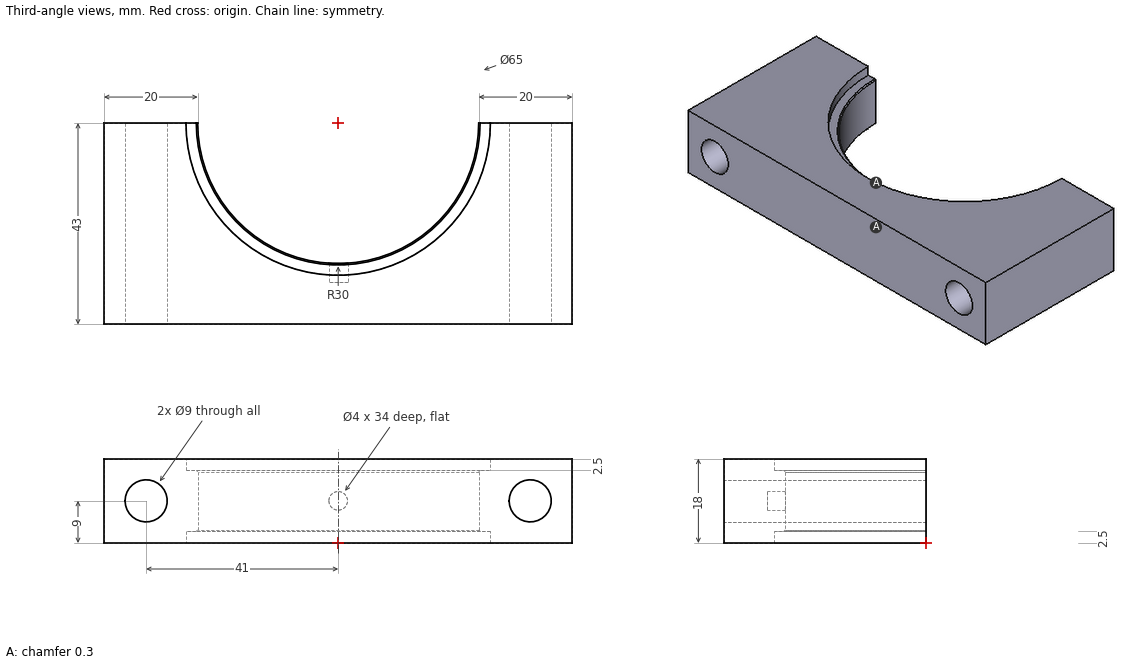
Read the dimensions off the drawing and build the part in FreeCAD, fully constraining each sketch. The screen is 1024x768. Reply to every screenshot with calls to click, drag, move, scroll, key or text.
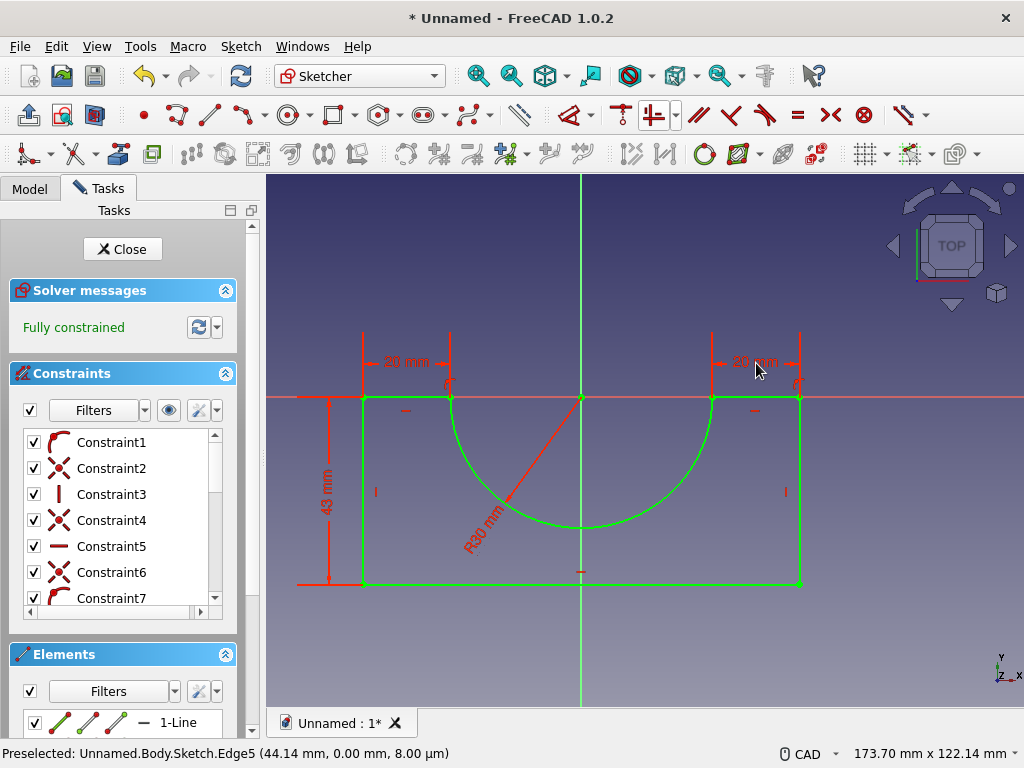
click(123, 249)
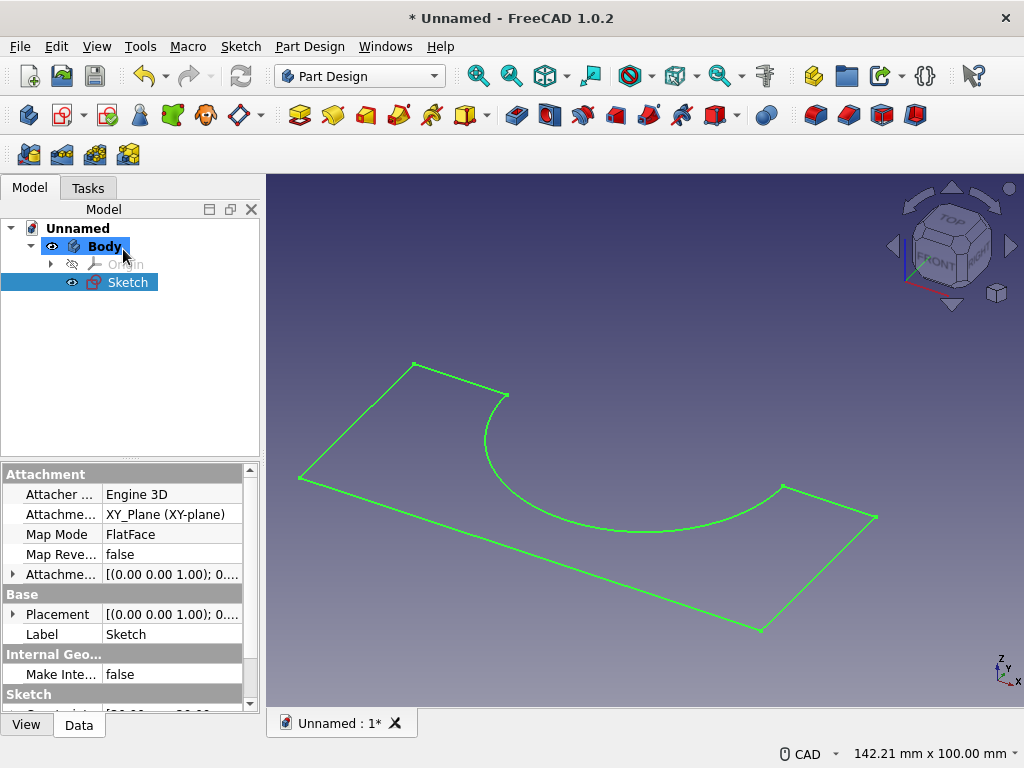
click(300, 116)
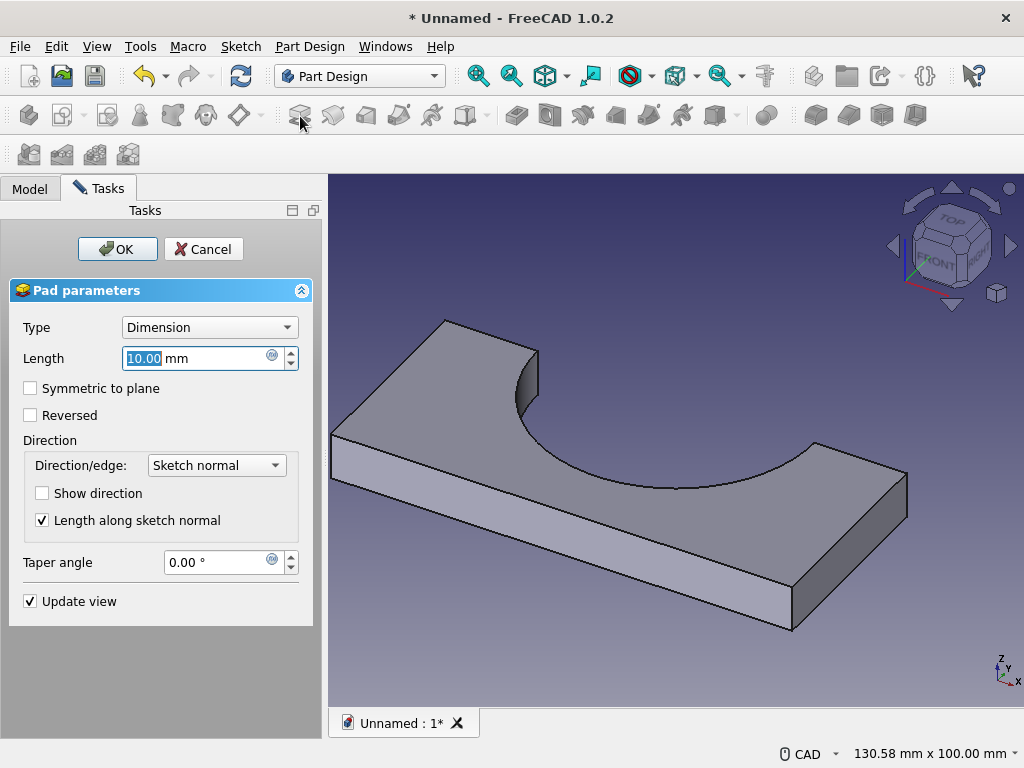
text(18)
key(Tab)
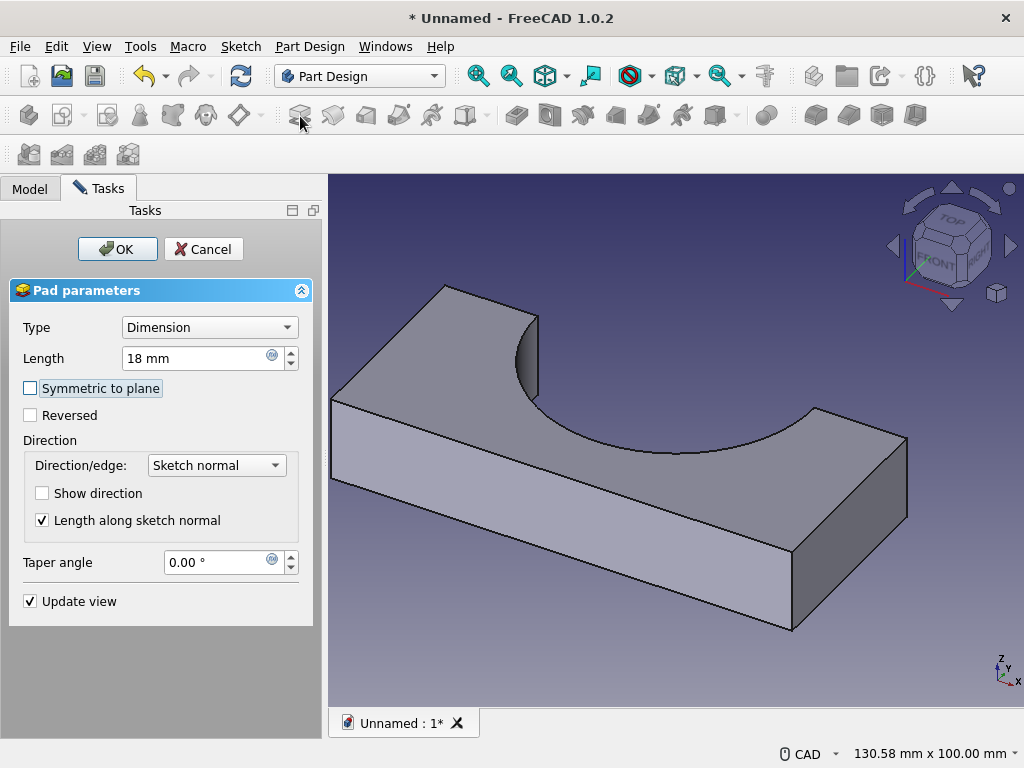
click(118, 249)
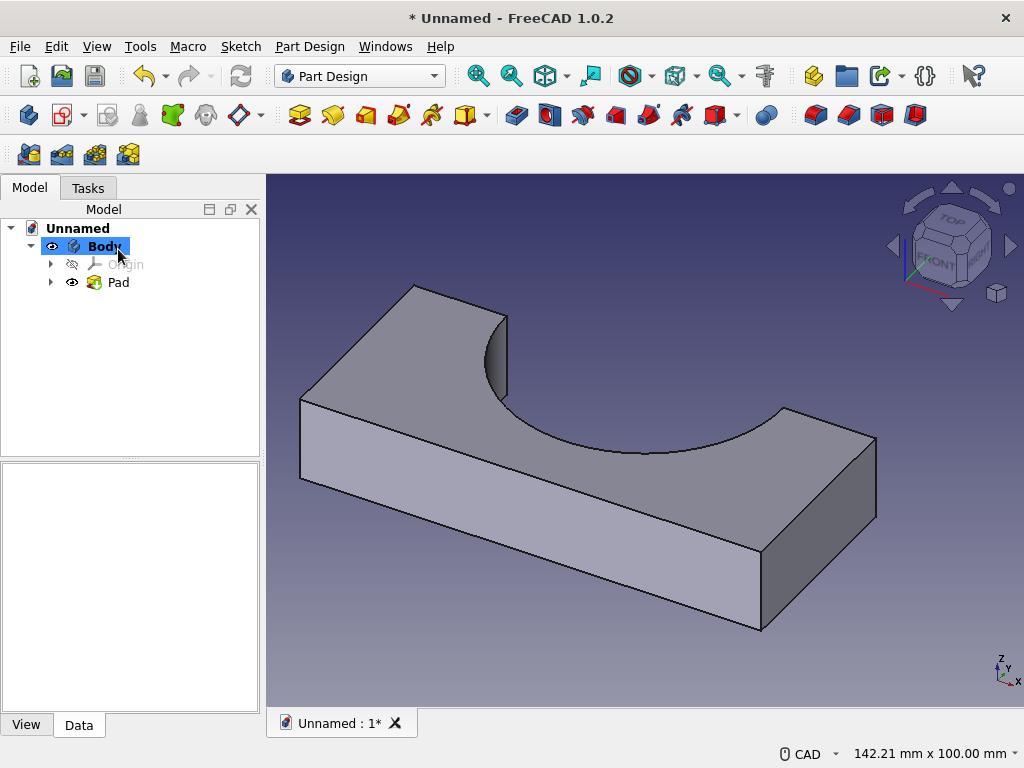
click(439, 390)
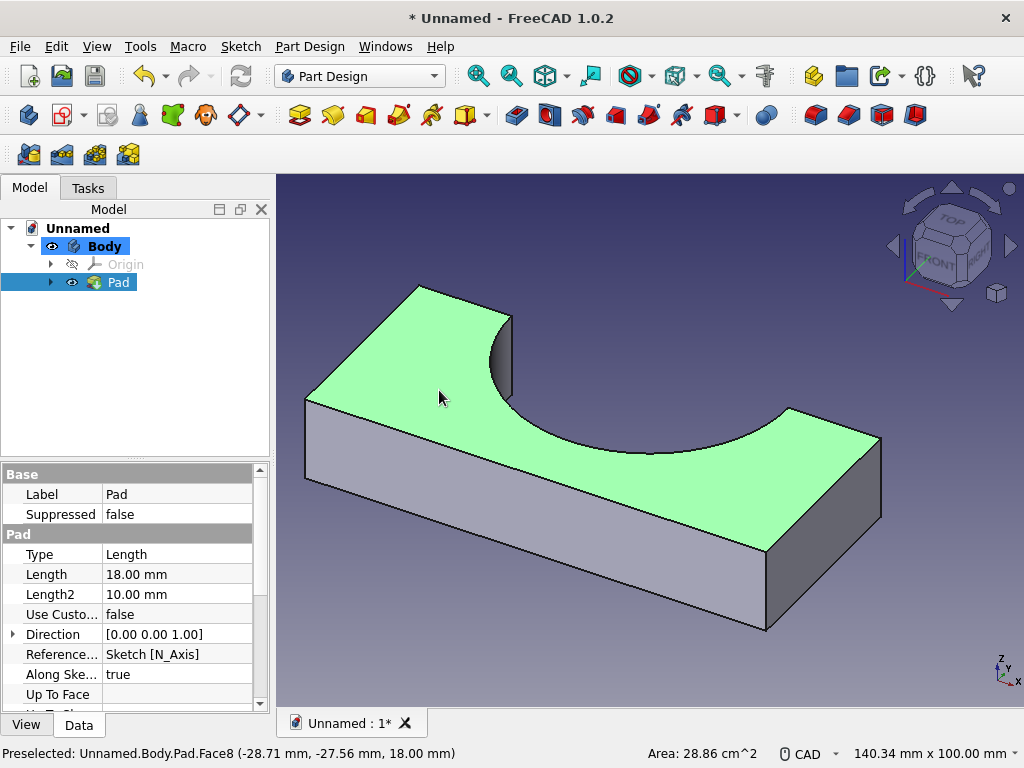
click(62, 116)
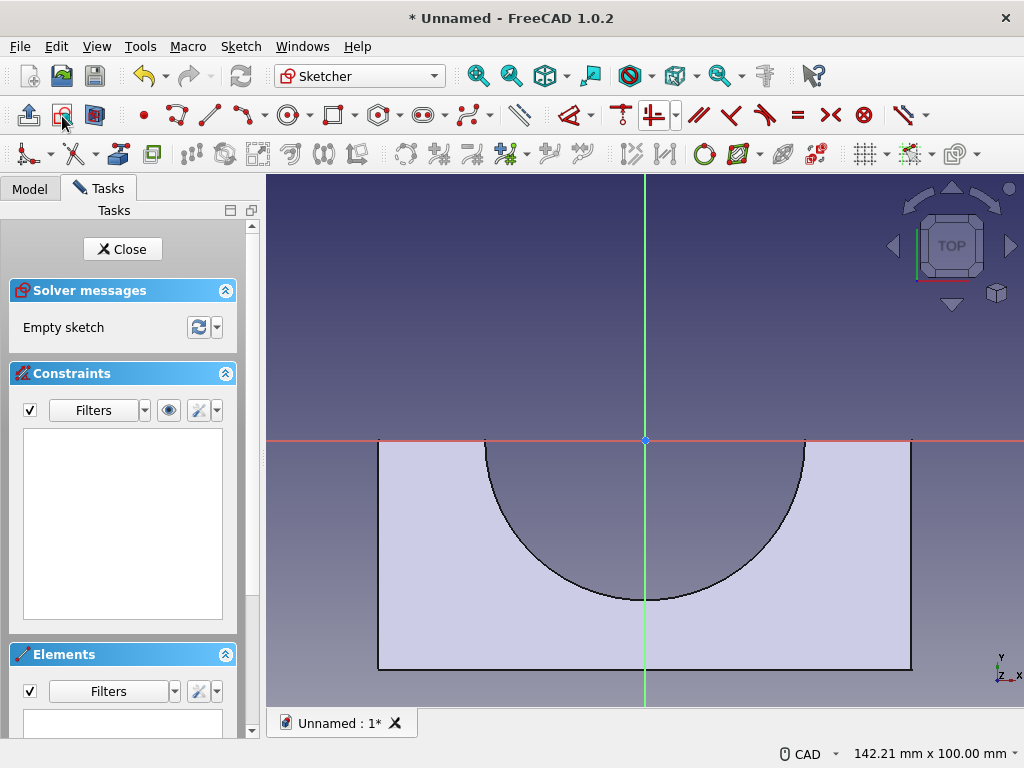
click(288, 116)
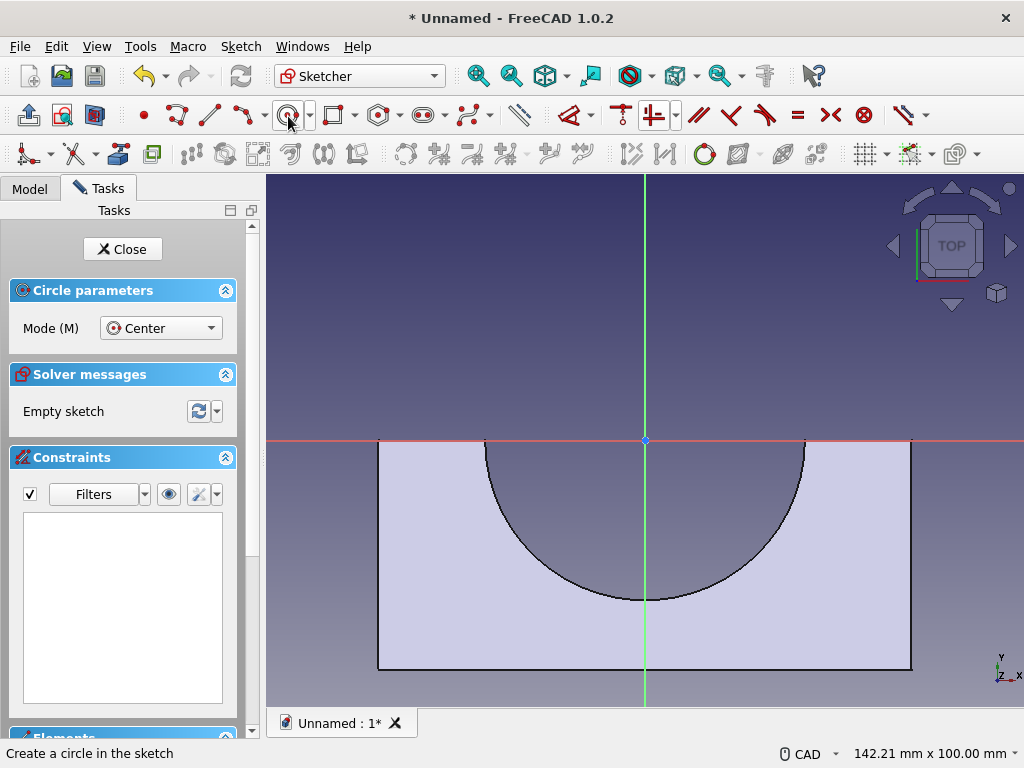
click(645, 440)
move(767, 318)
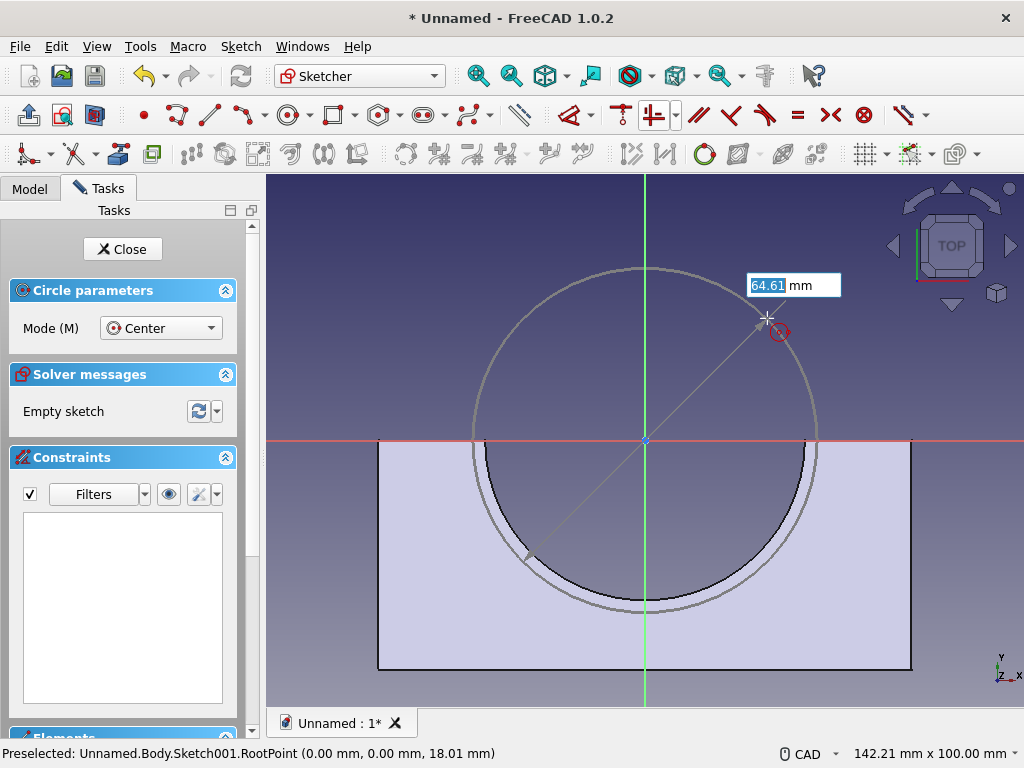
text(65)
key(Return)
key(Escape)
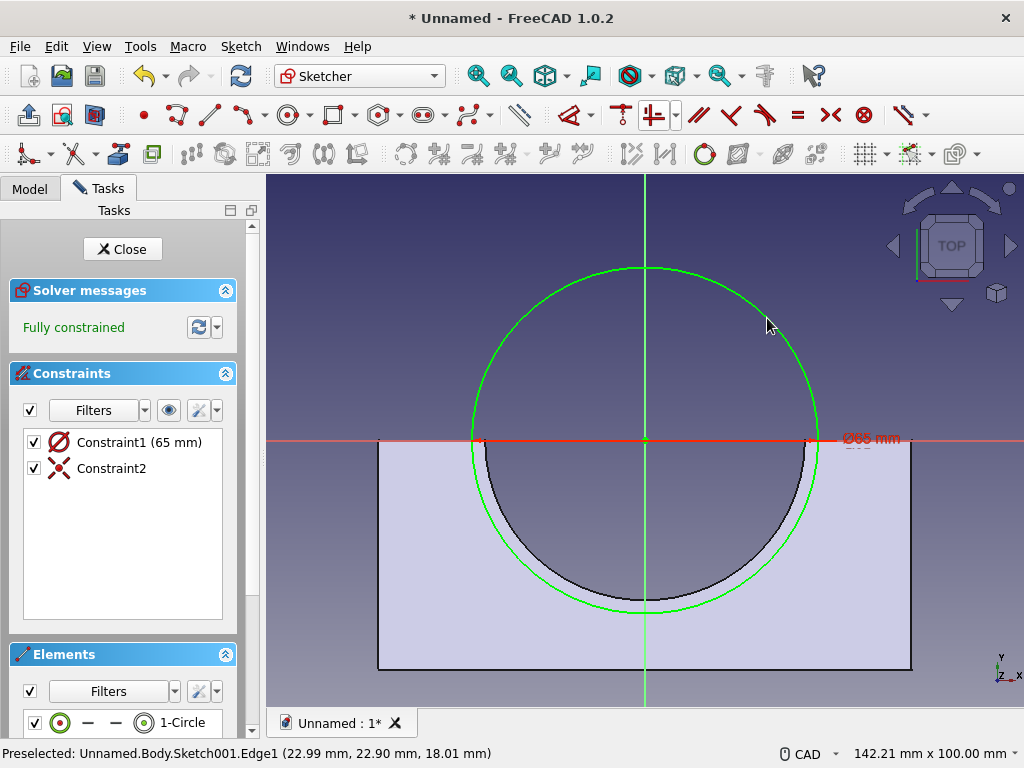
click(123, 249)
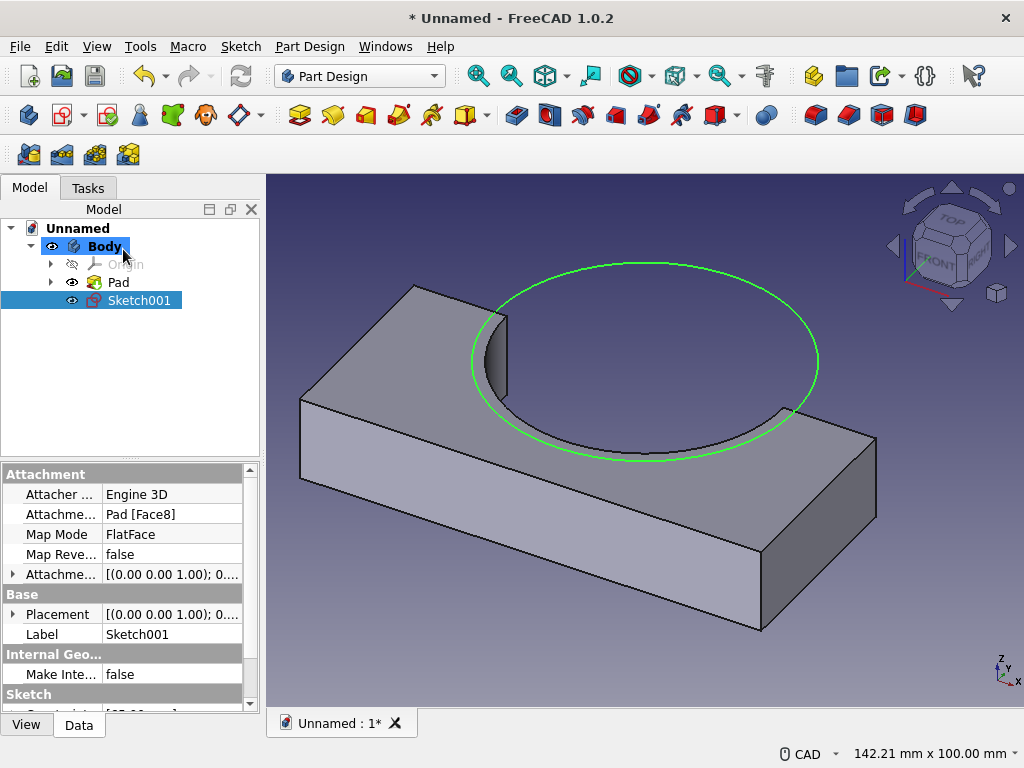
click(517, 116)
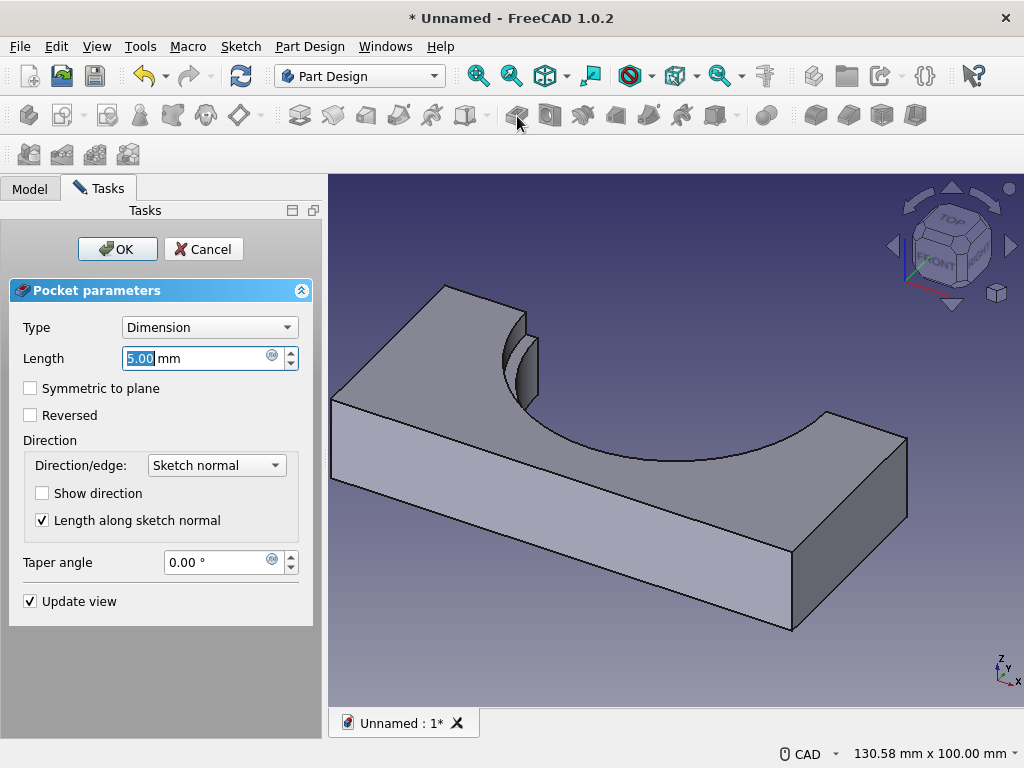
text(2.5)
key(Tab)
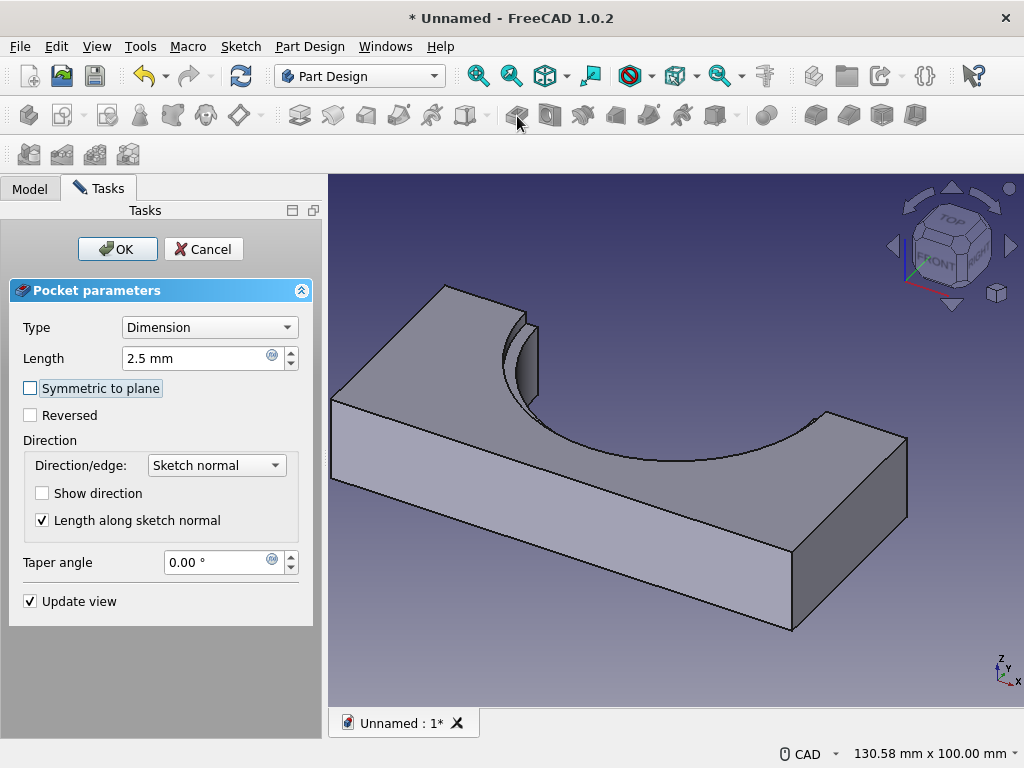
click(118, 249)